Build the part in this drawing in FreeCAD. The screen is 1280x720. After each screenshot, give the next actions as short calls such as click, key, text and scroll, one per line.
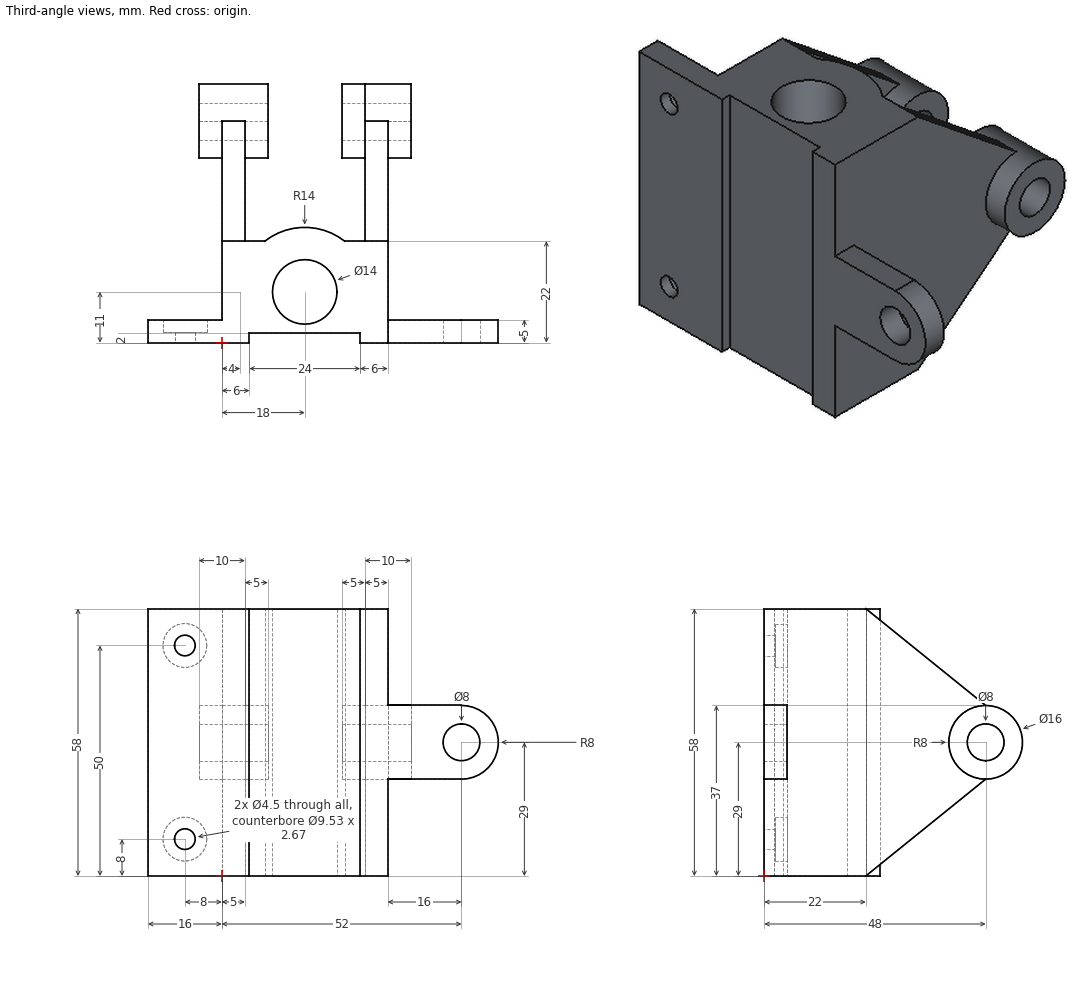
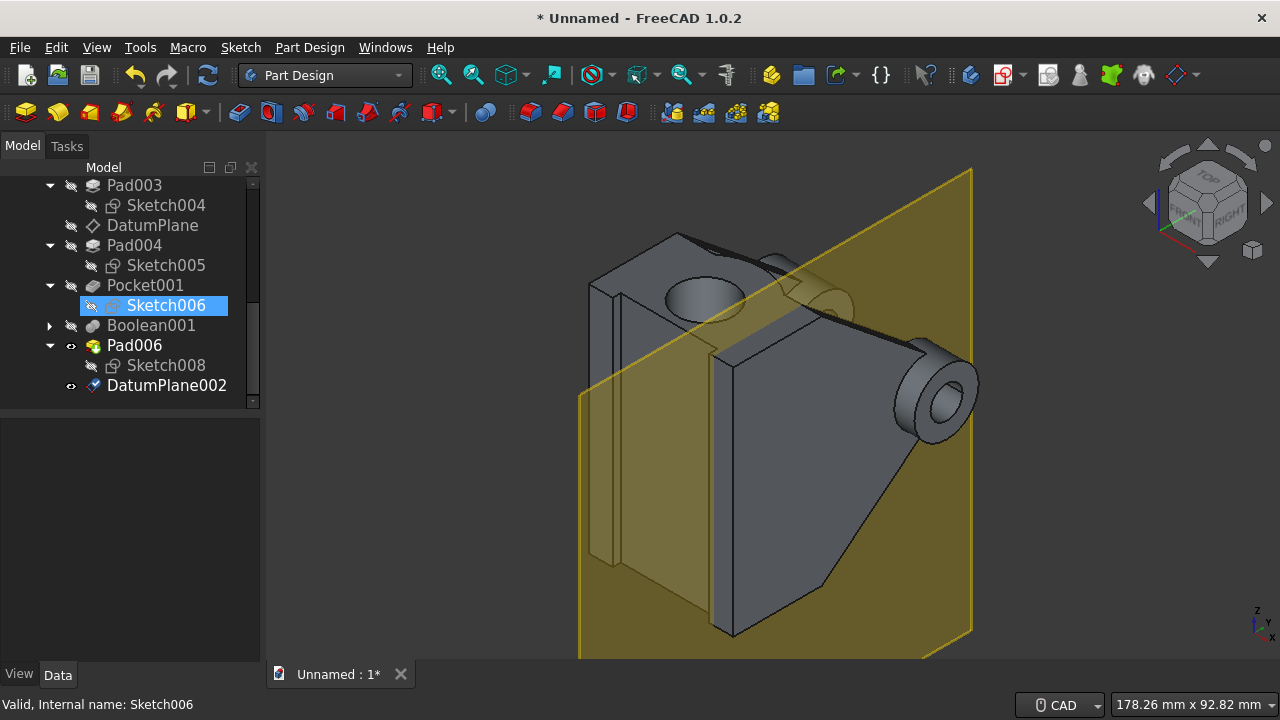
click(116, 386)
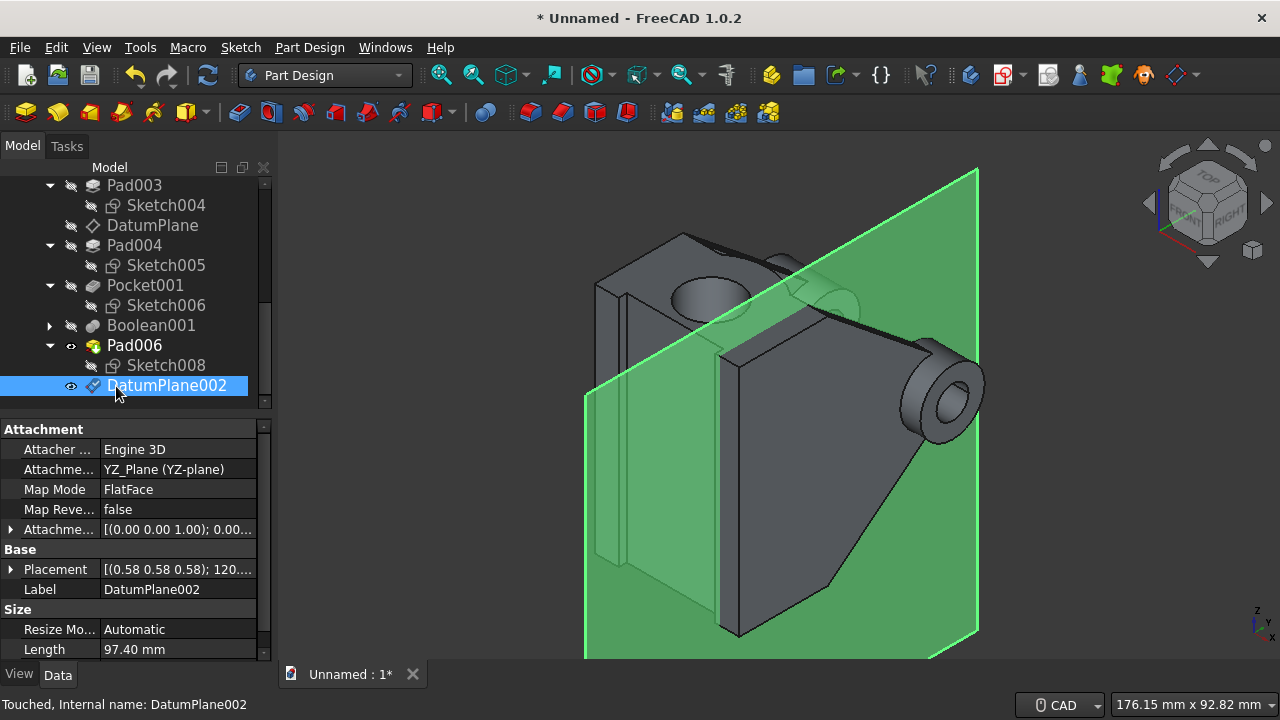
click(1004, 76)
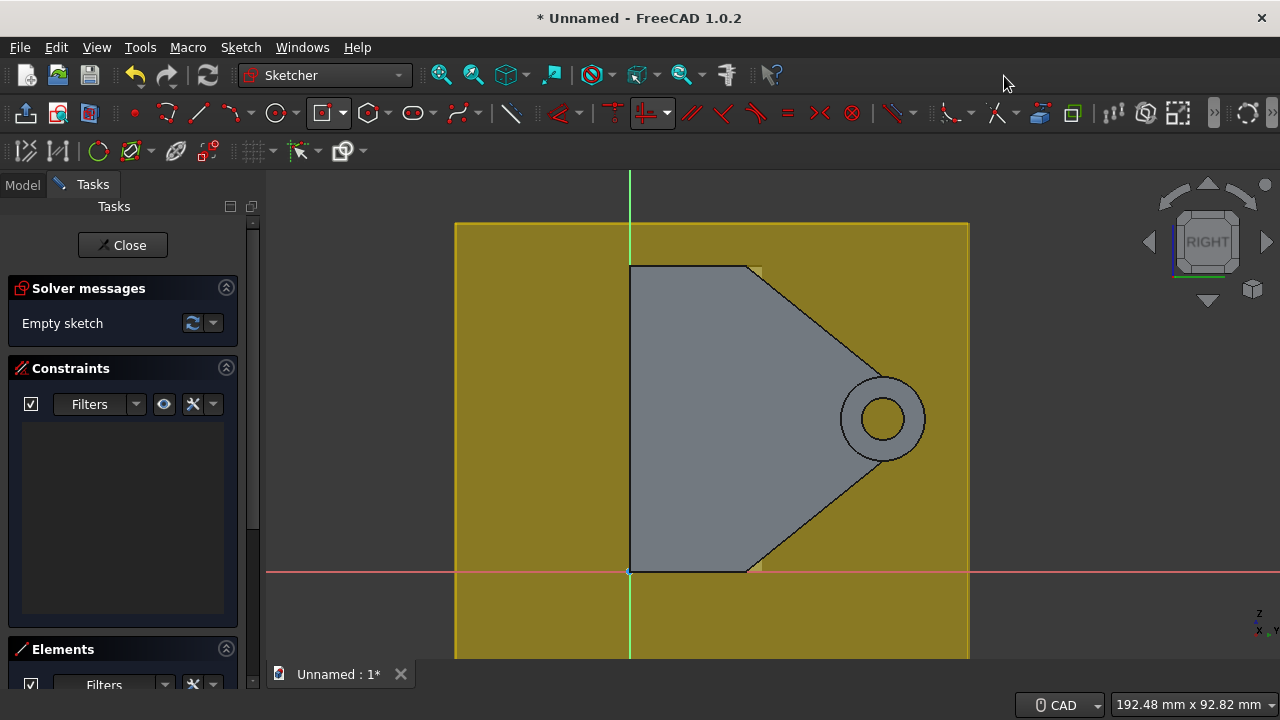
key(q)
key(s)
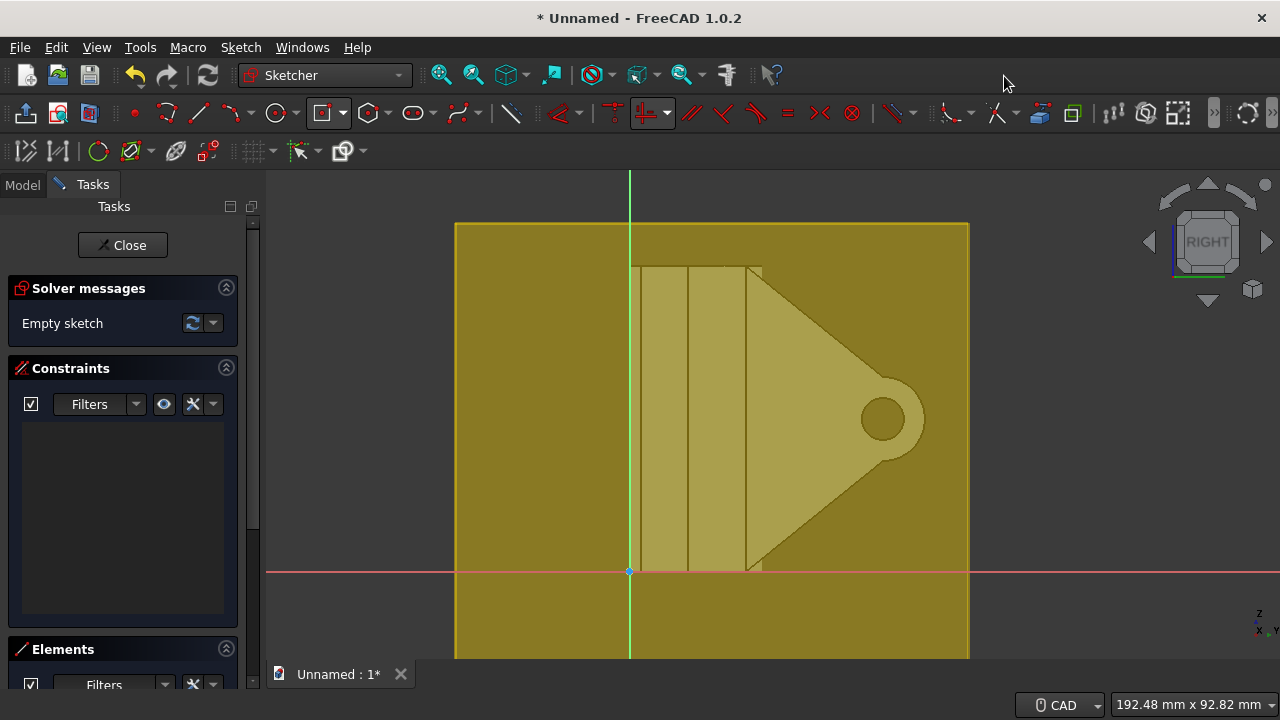
scroll(960, 421, up, 6)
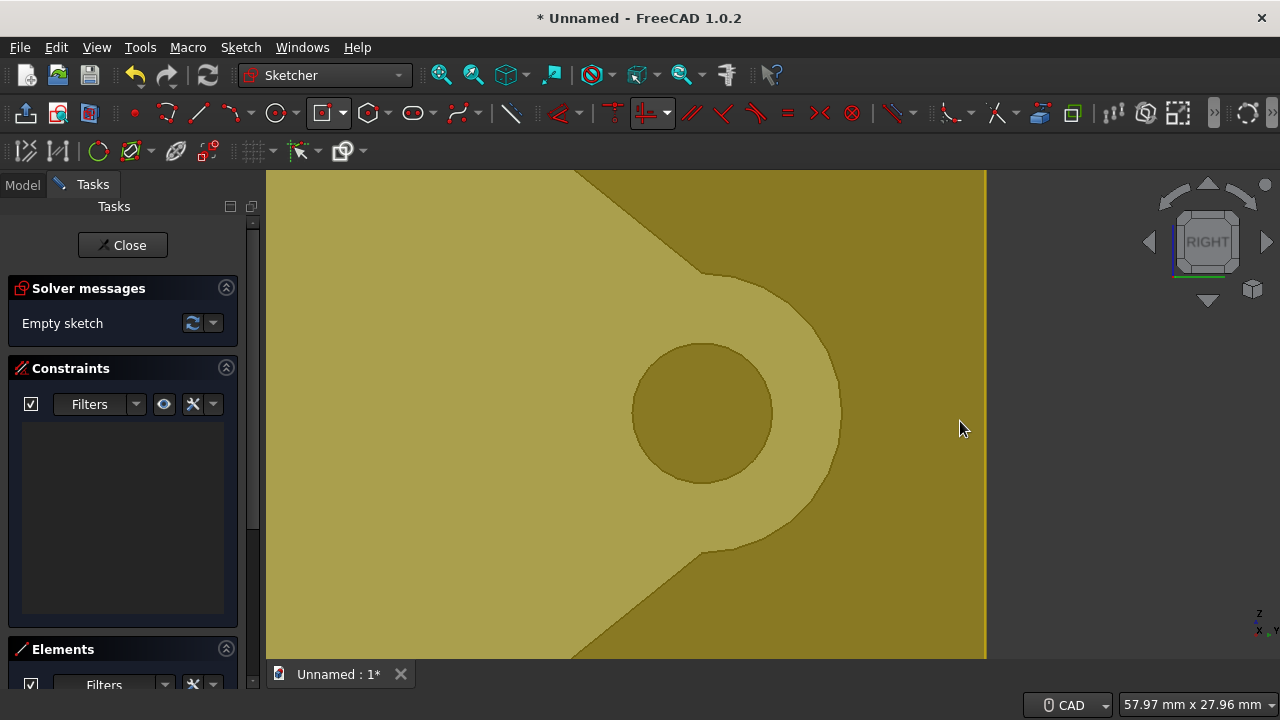
key(g)
key(c)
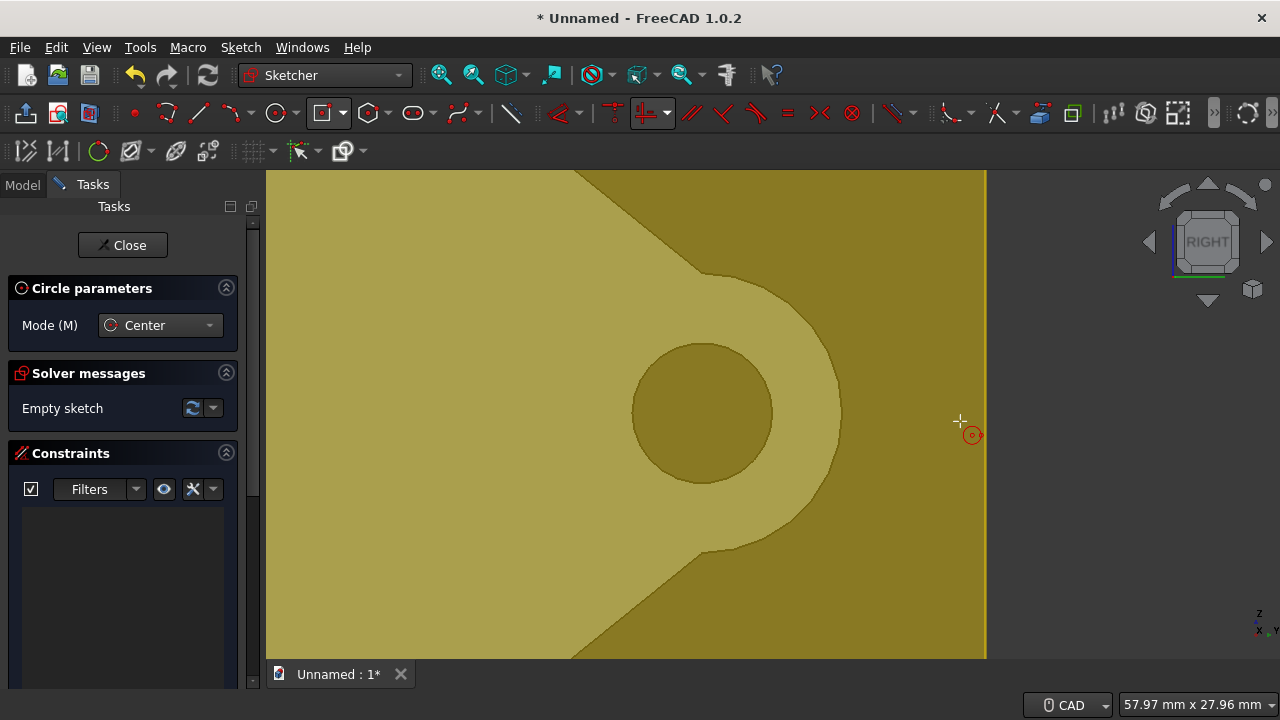
click(702, 413)
move(801, 314)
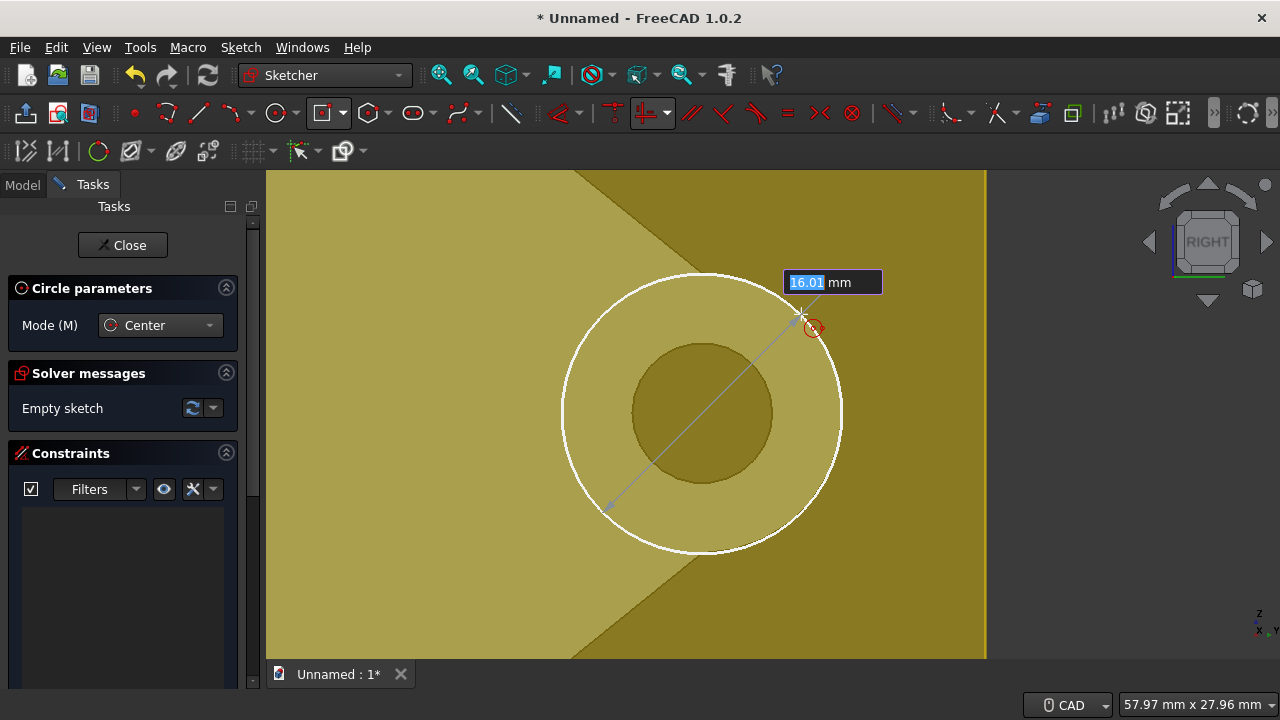
text(16)
key(Return)
key(Escape)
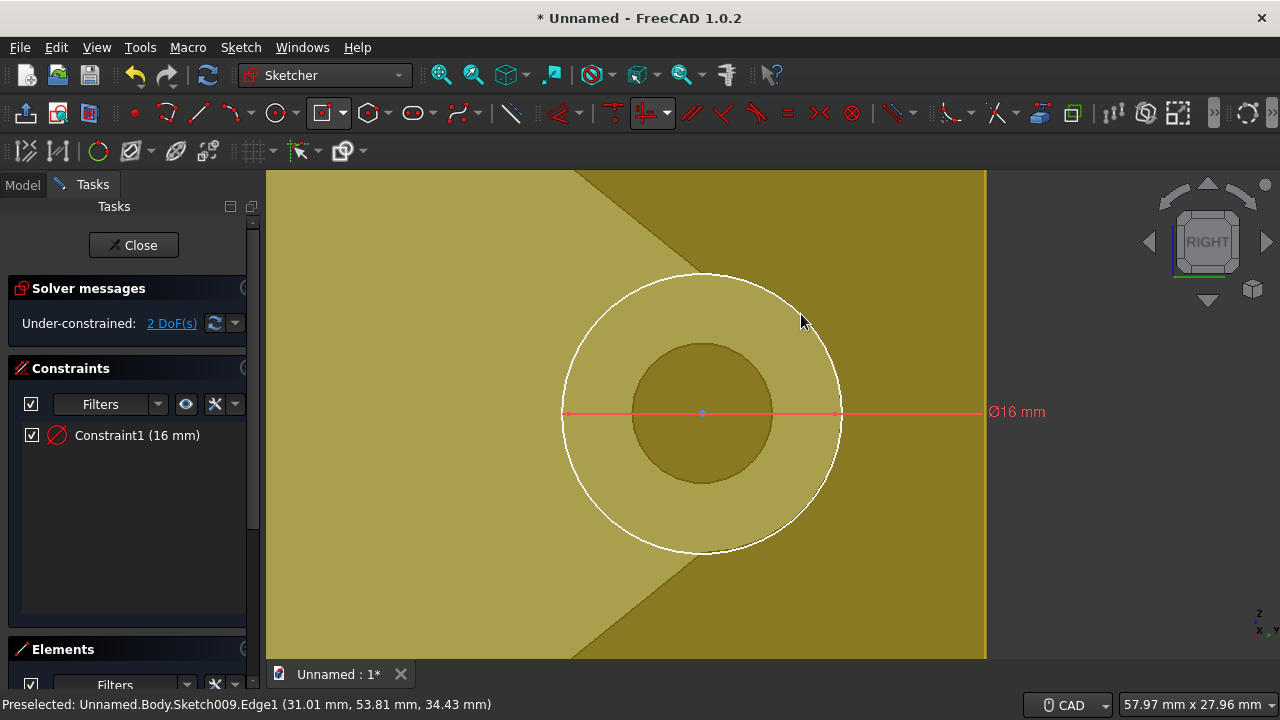
key(d)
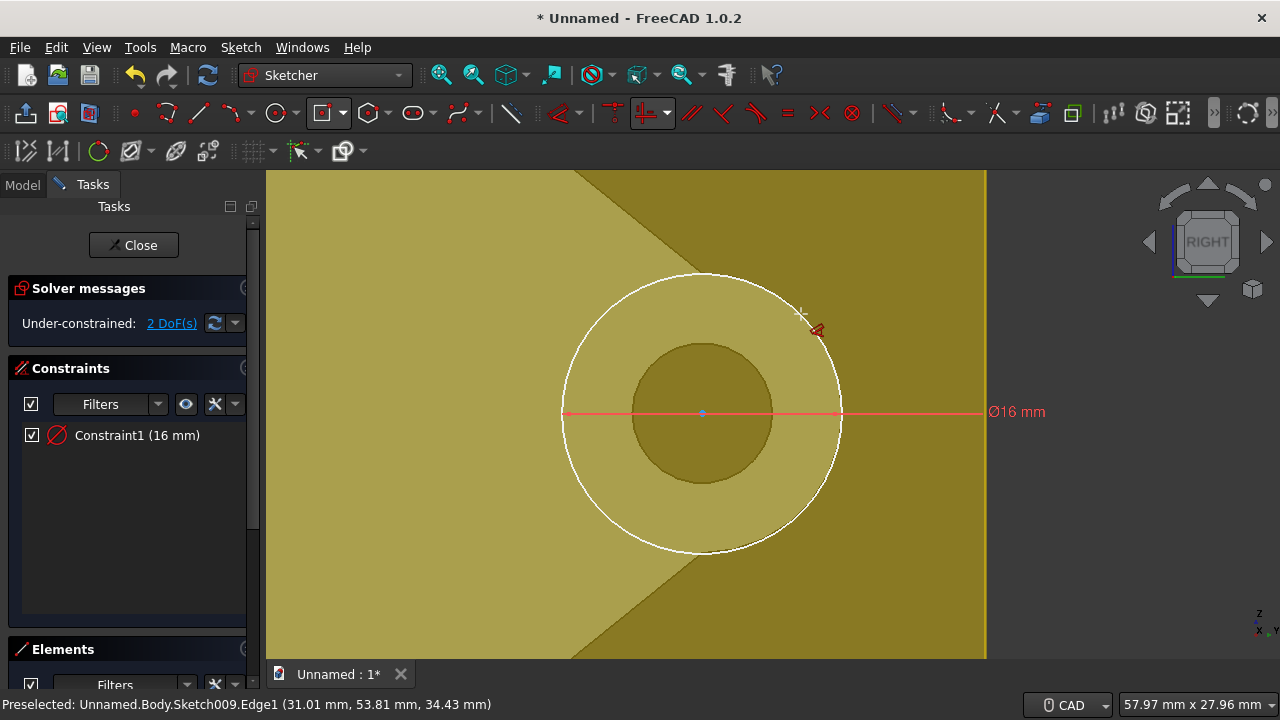
click(702, 414)
click(498, 380)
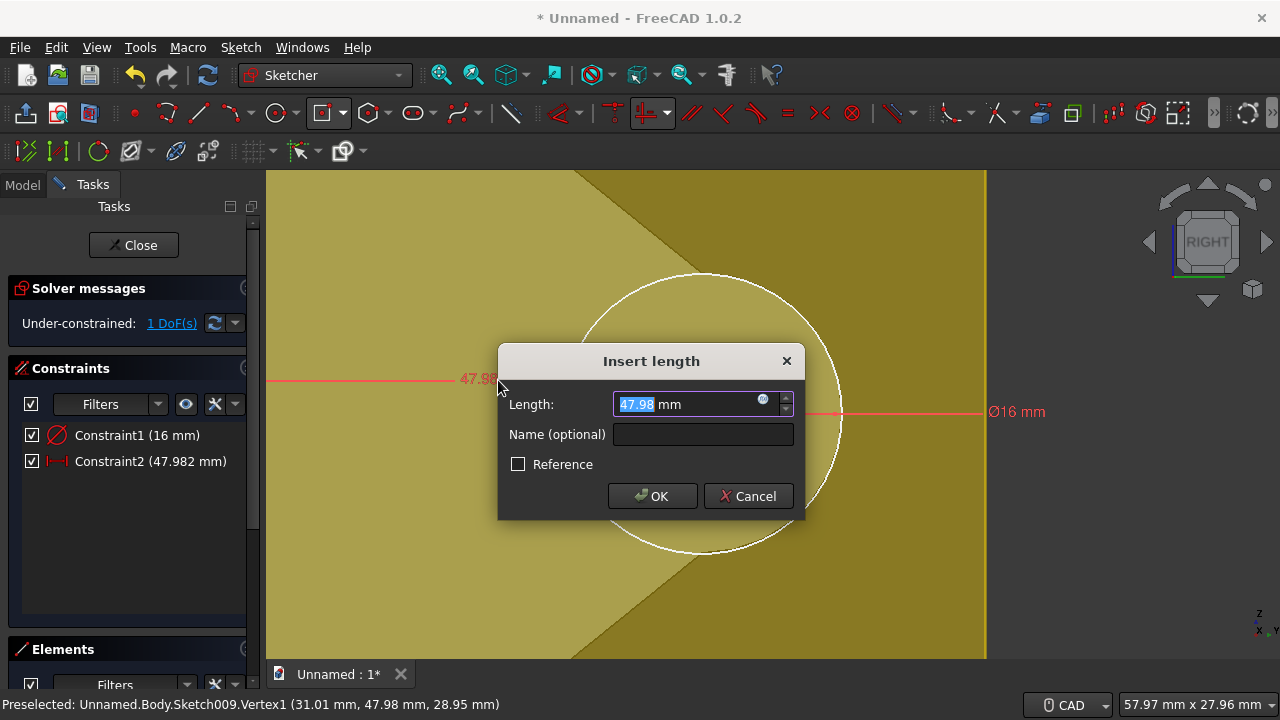
text(48)
key(Return)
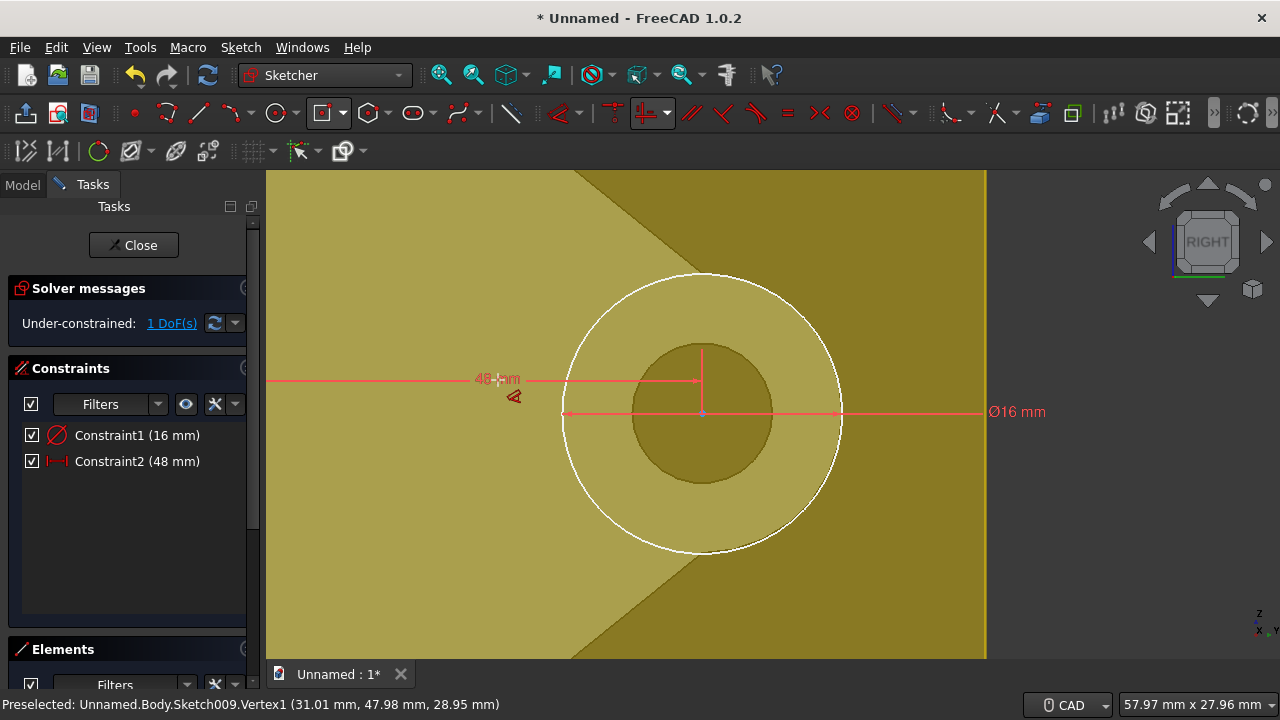
click(702, 414)
click(736, 522)